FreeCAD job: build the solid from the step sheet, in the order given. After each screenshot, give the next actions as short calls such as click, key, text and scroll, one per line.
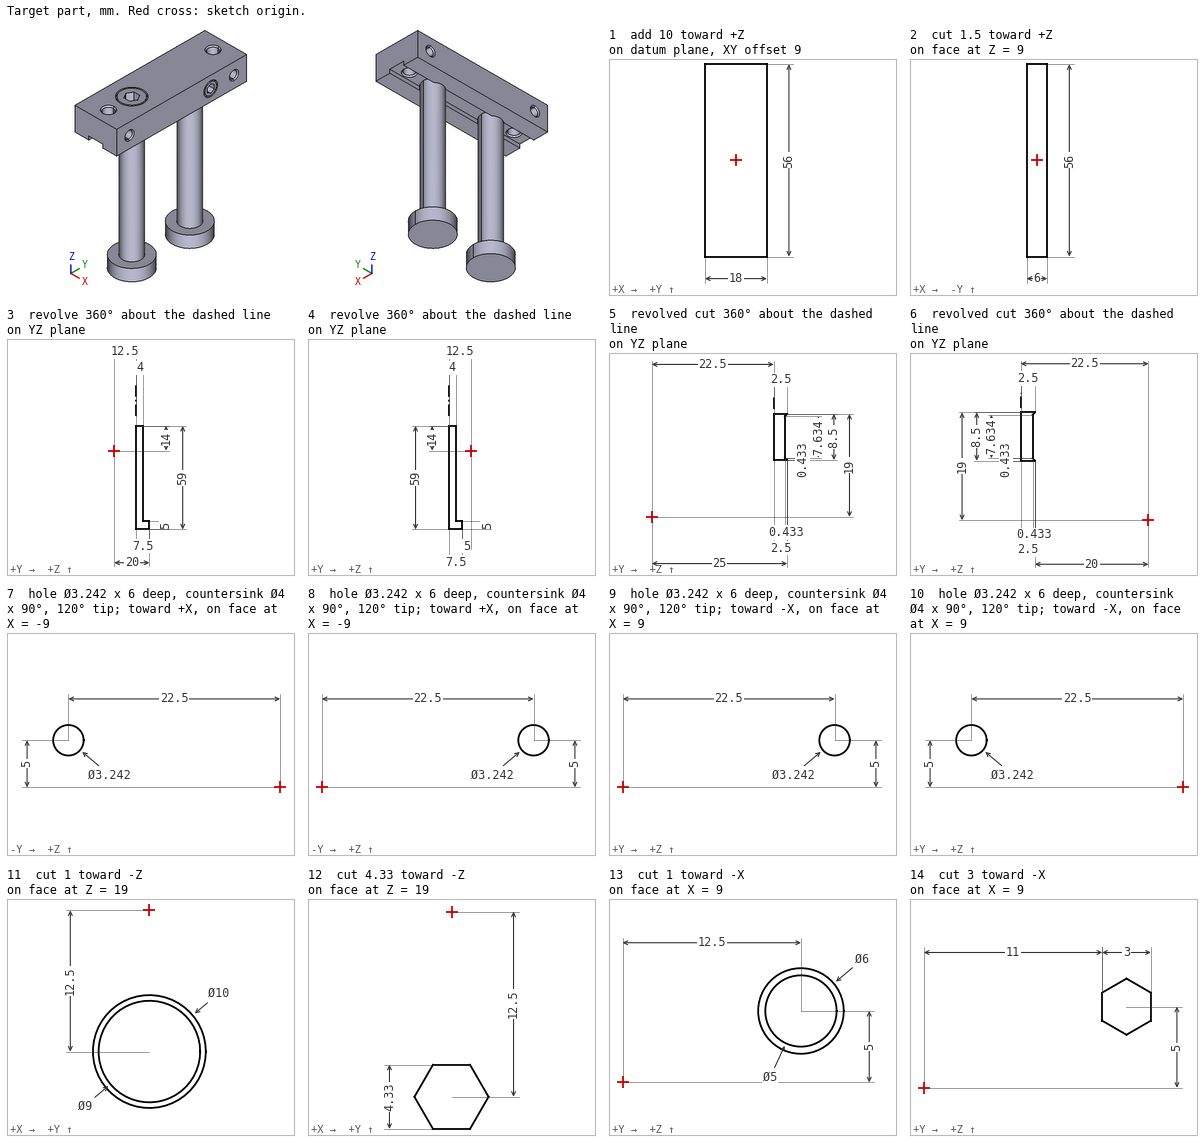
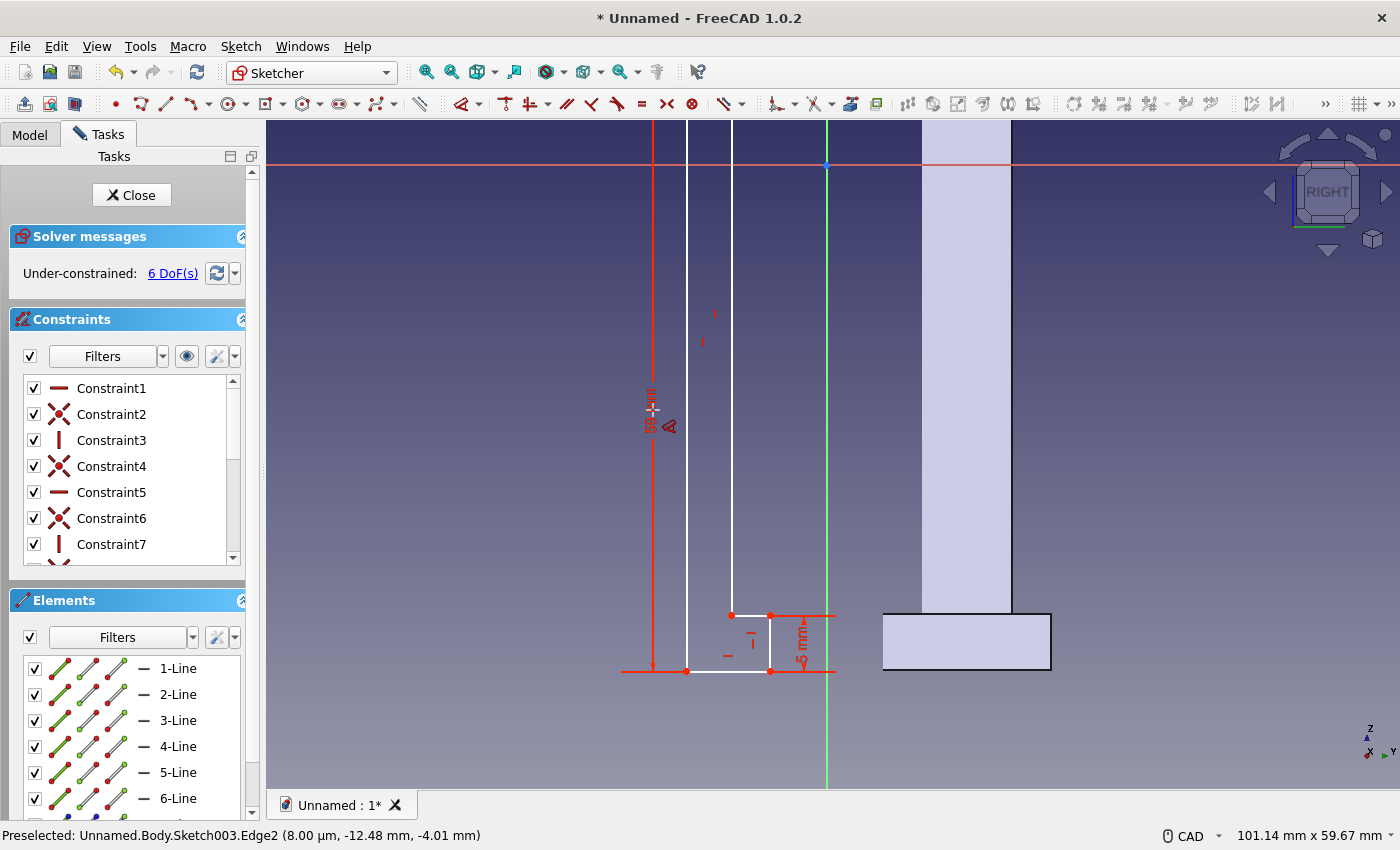
click(770, 672)
click(799, 706)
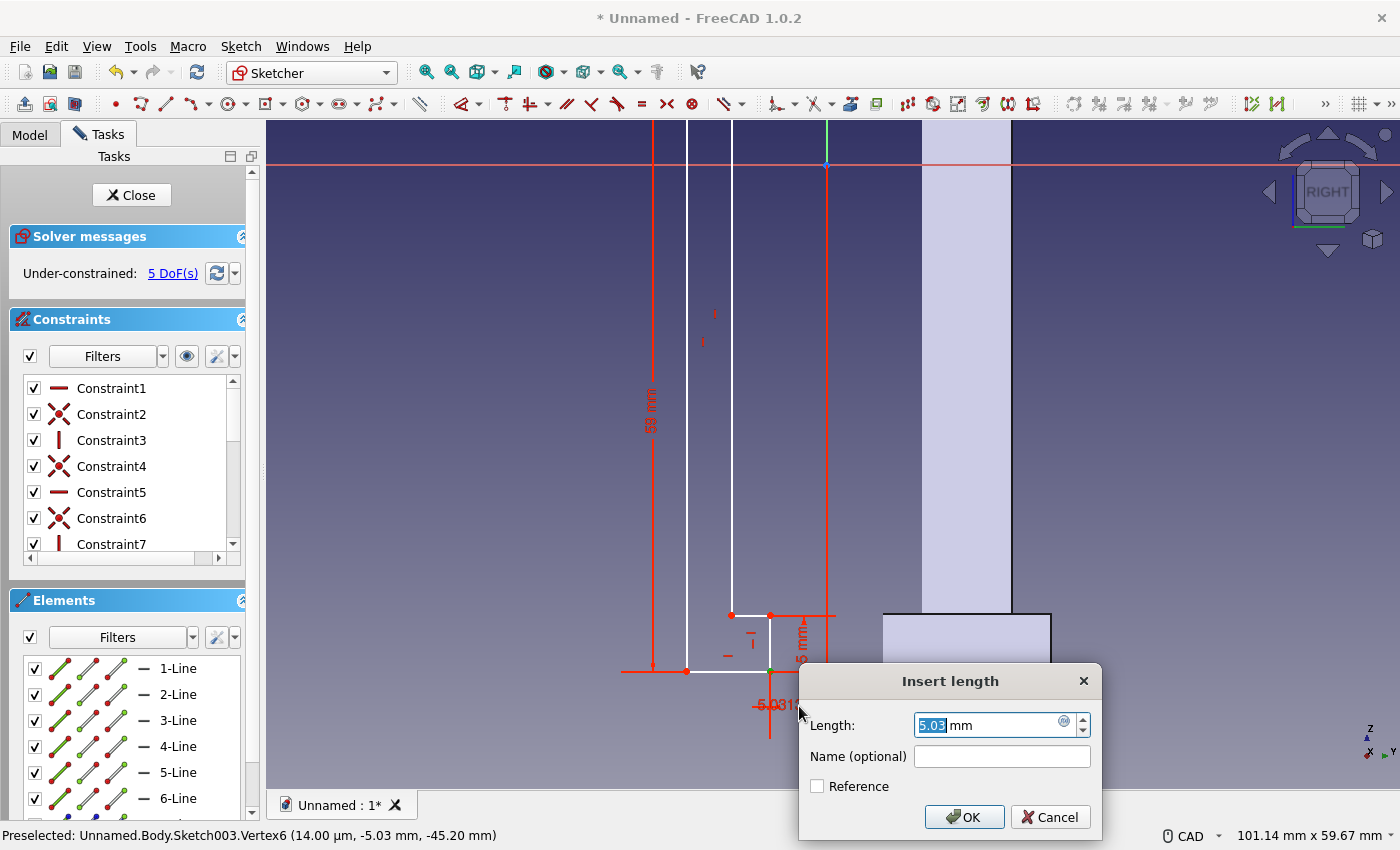
text(5)
key(Return)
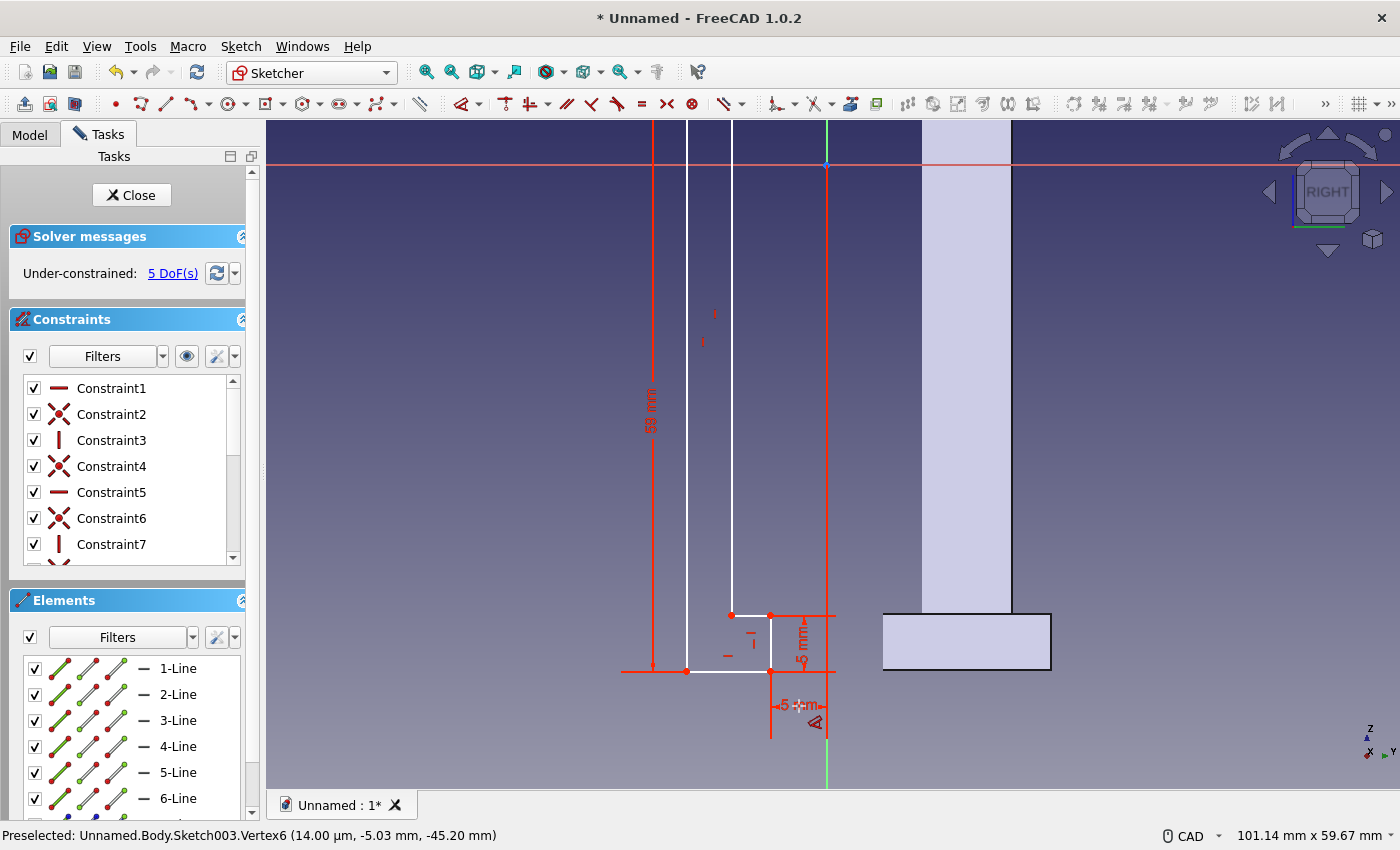
click(712, 672)
click(710, 706)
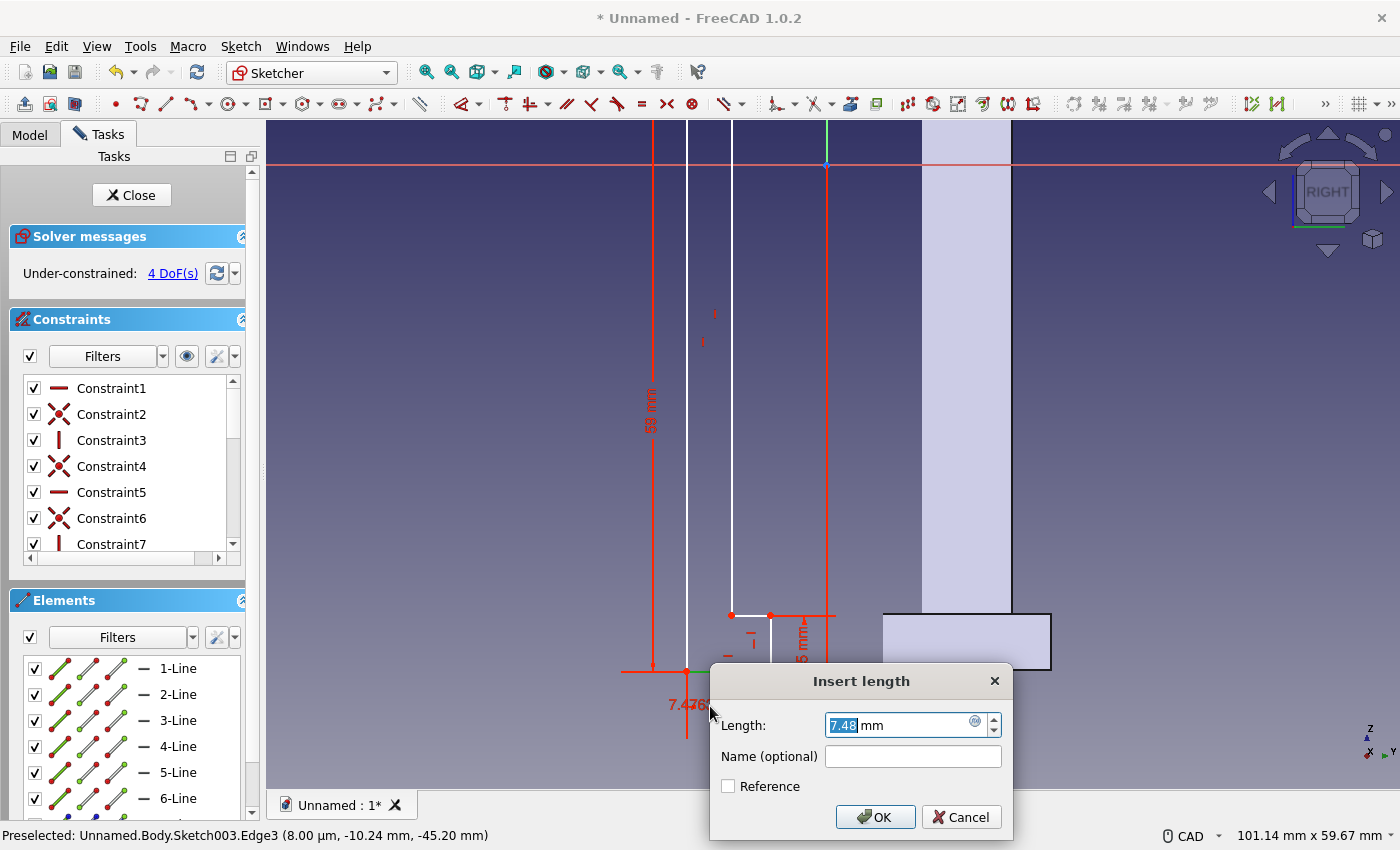
text(7.5)
key(Return)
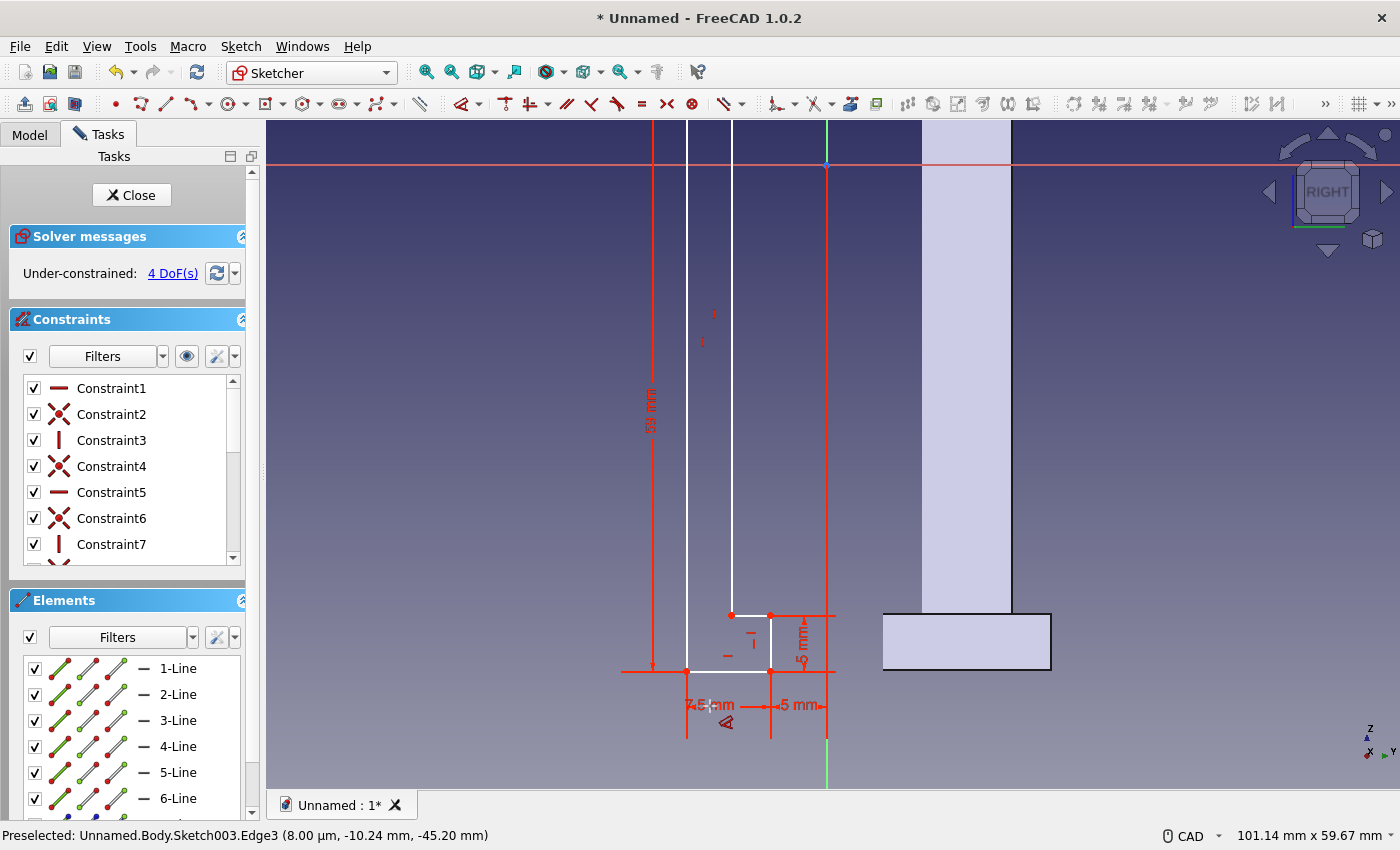
scroll(771, 657, down, 4)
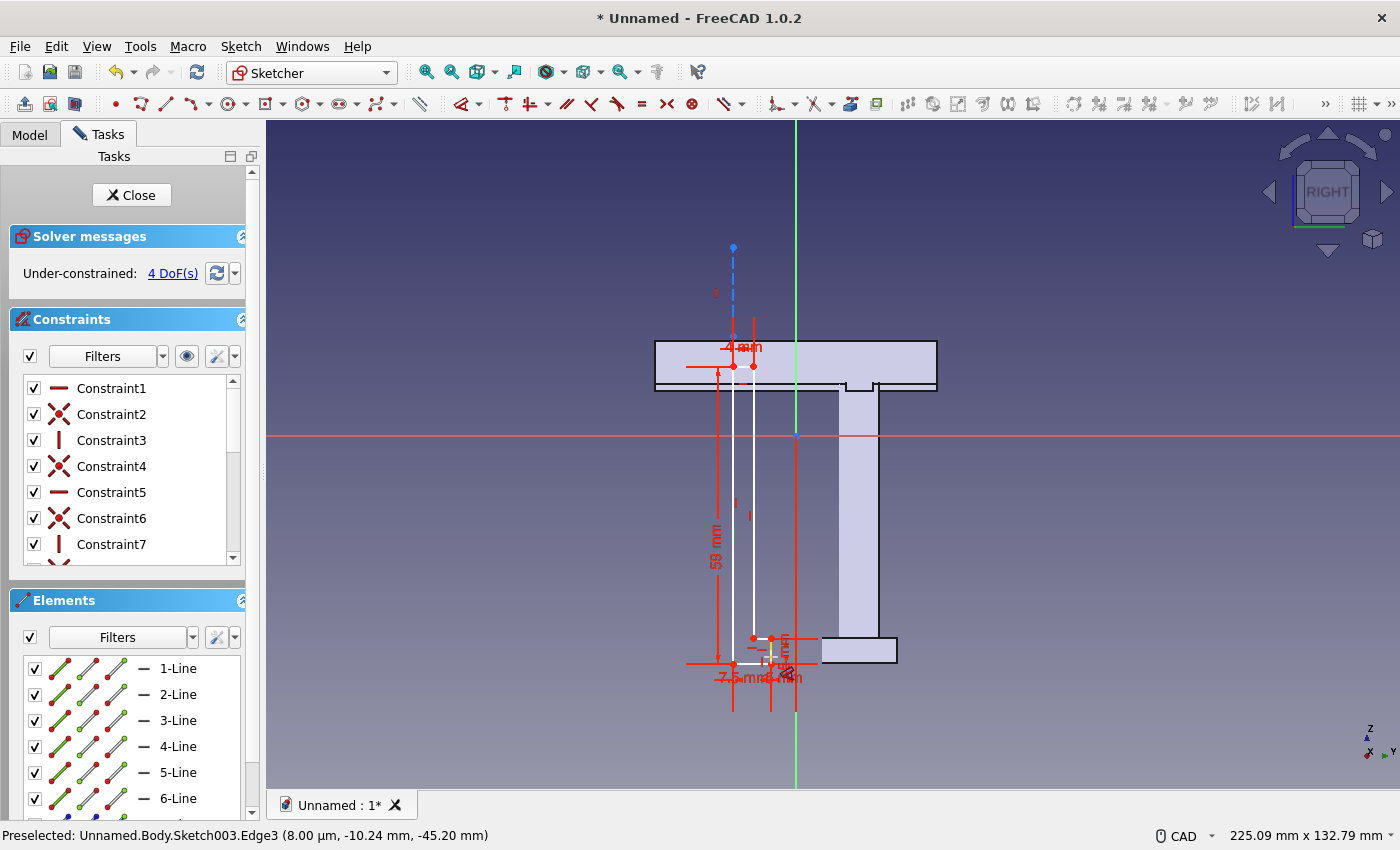
click(754, 367)
click(830, 402)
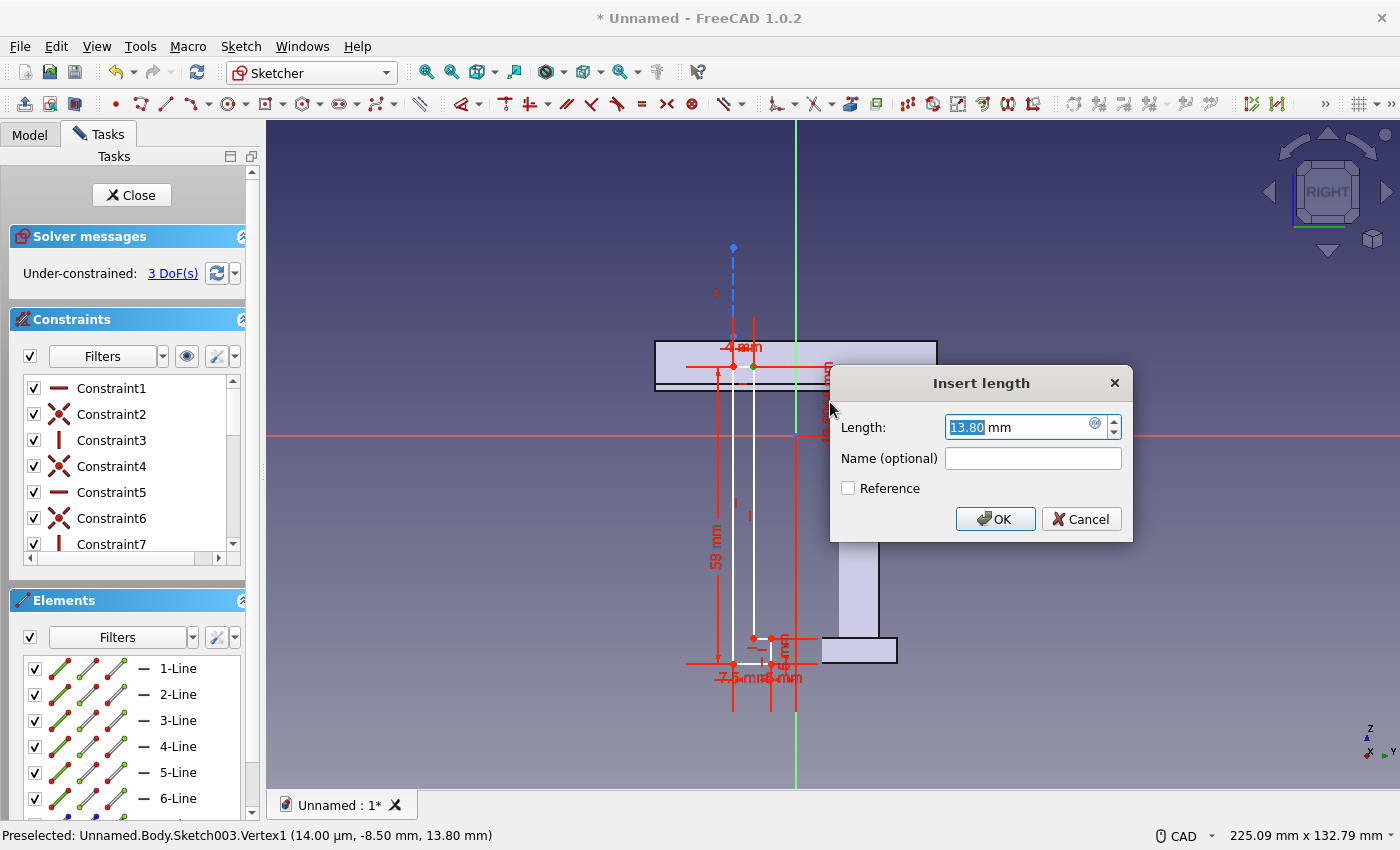
text(14)
key(Return)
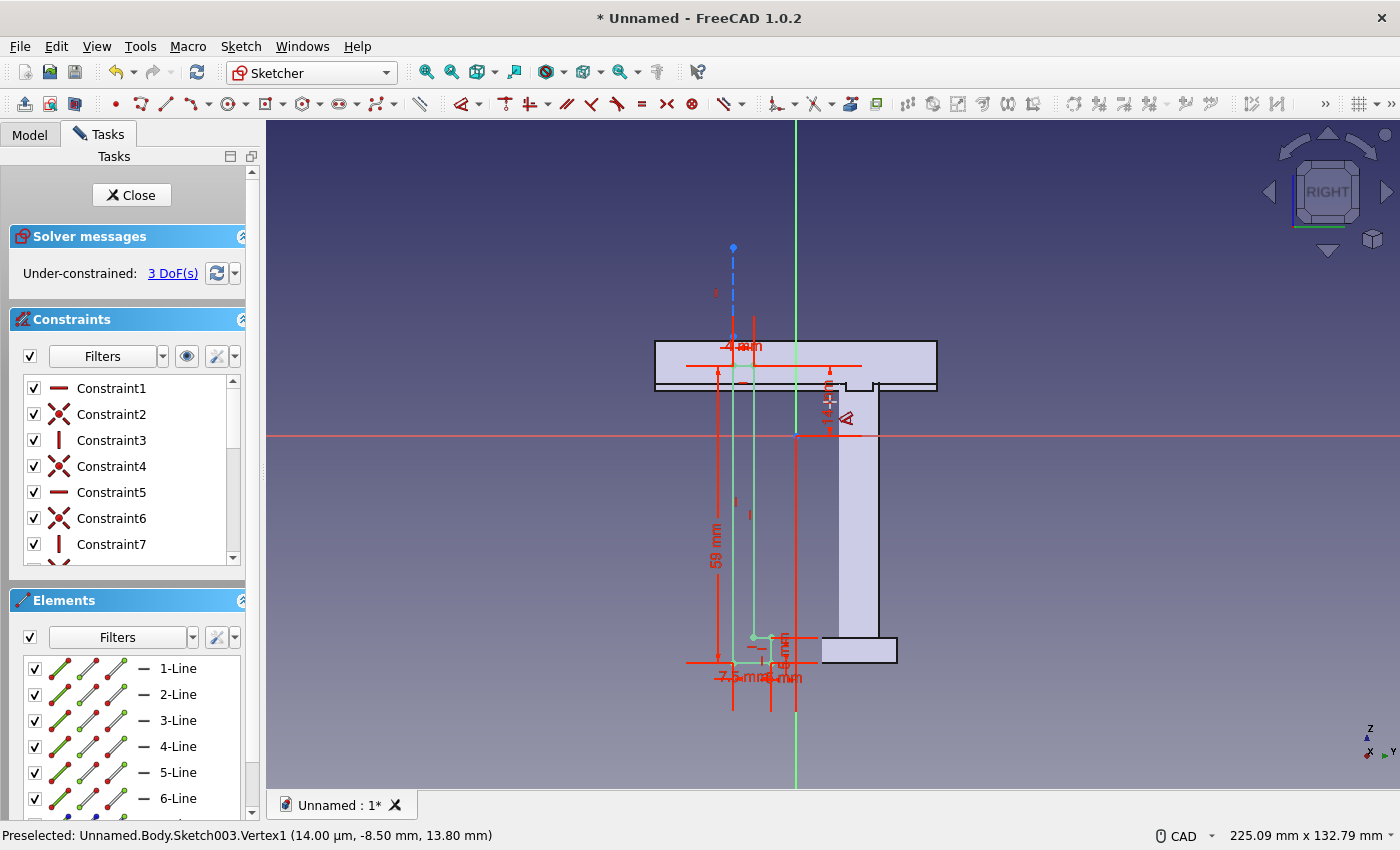
click(733, 337)
click(765, 303)